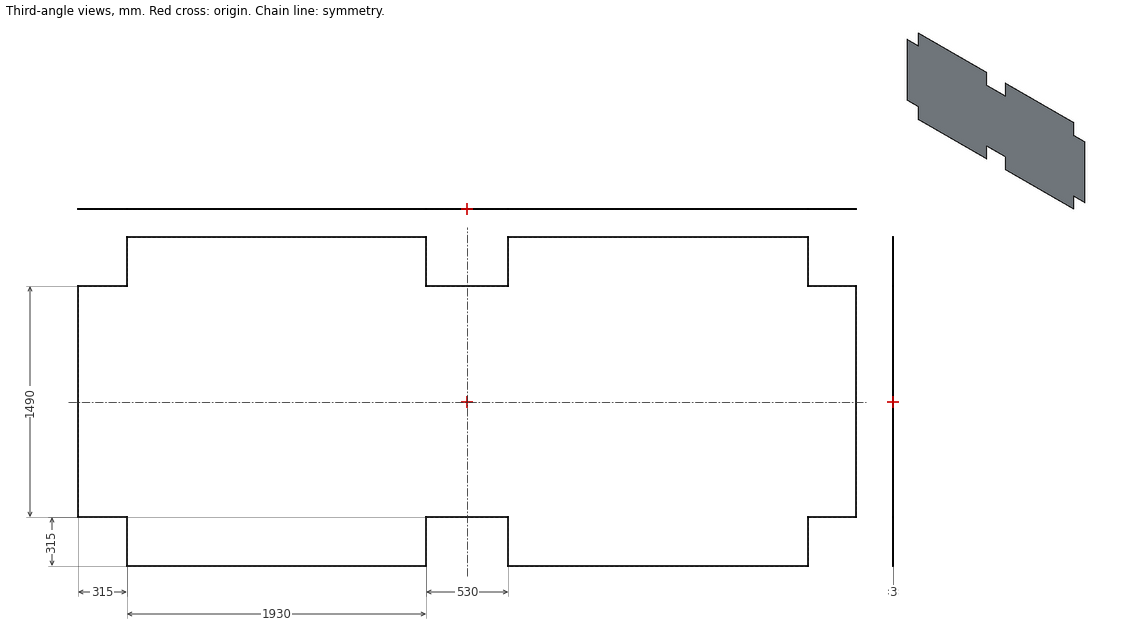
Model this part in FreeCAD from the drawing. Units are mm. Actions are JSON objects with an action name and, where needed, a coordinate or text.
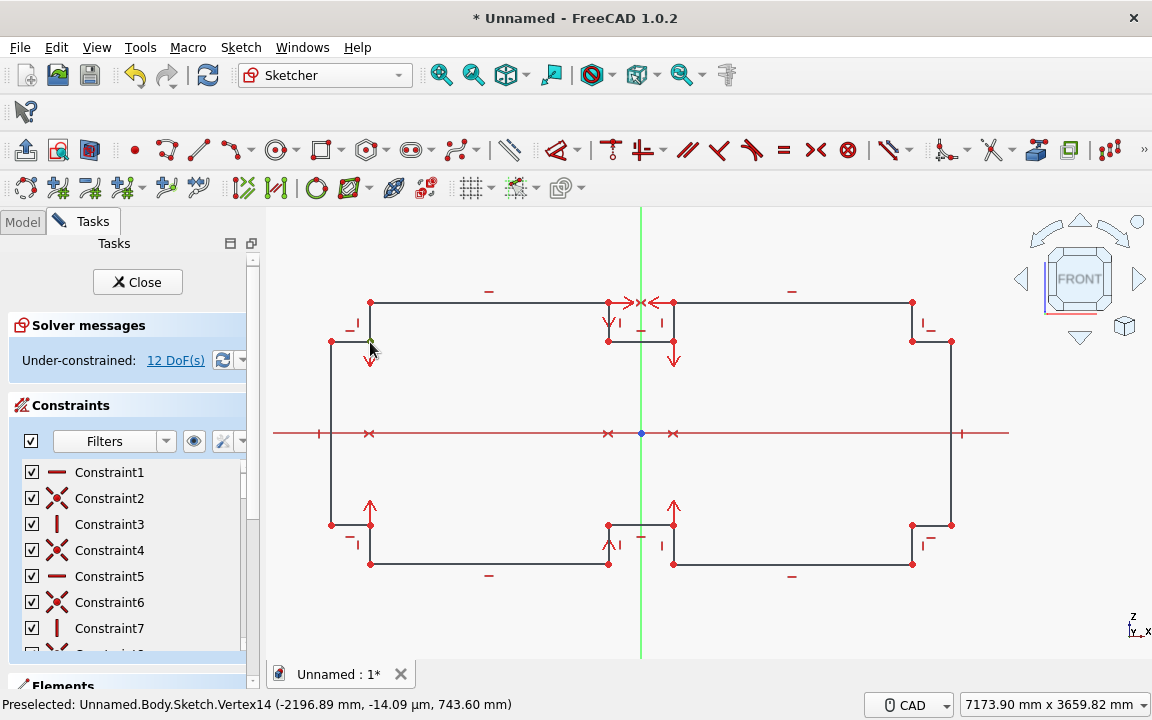
{"action": "left_click", "coordinate": [912, 342]}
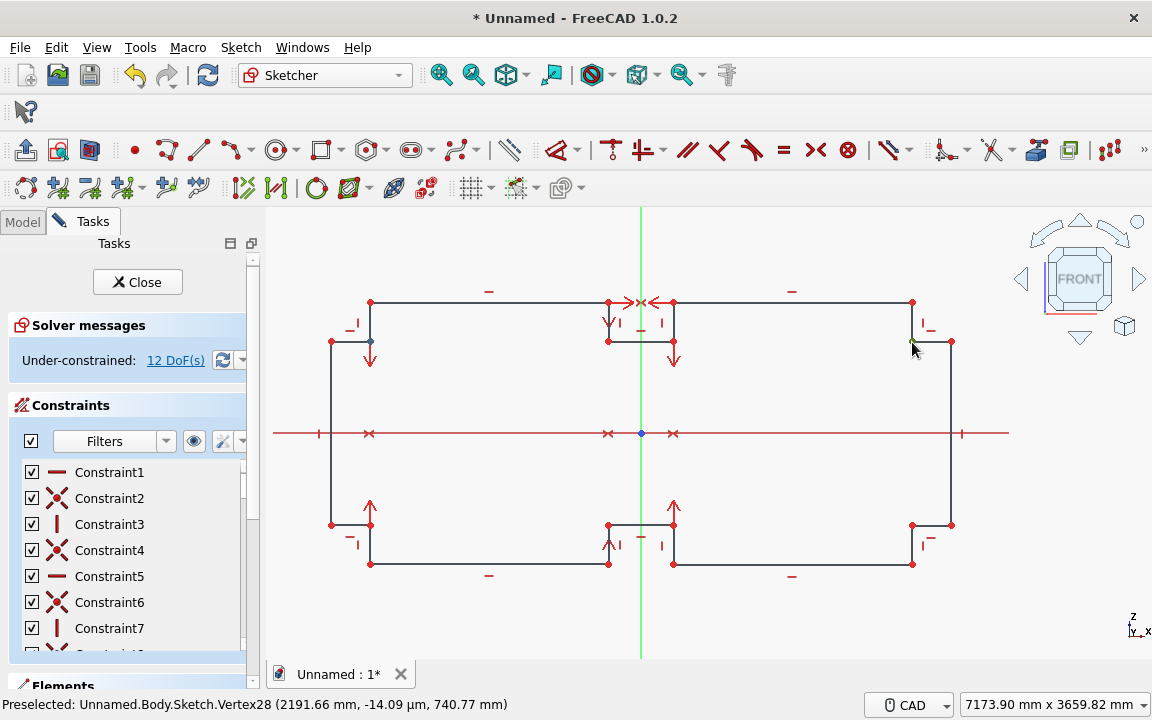
{"action": "left_click", "coordinate": [641, 603]}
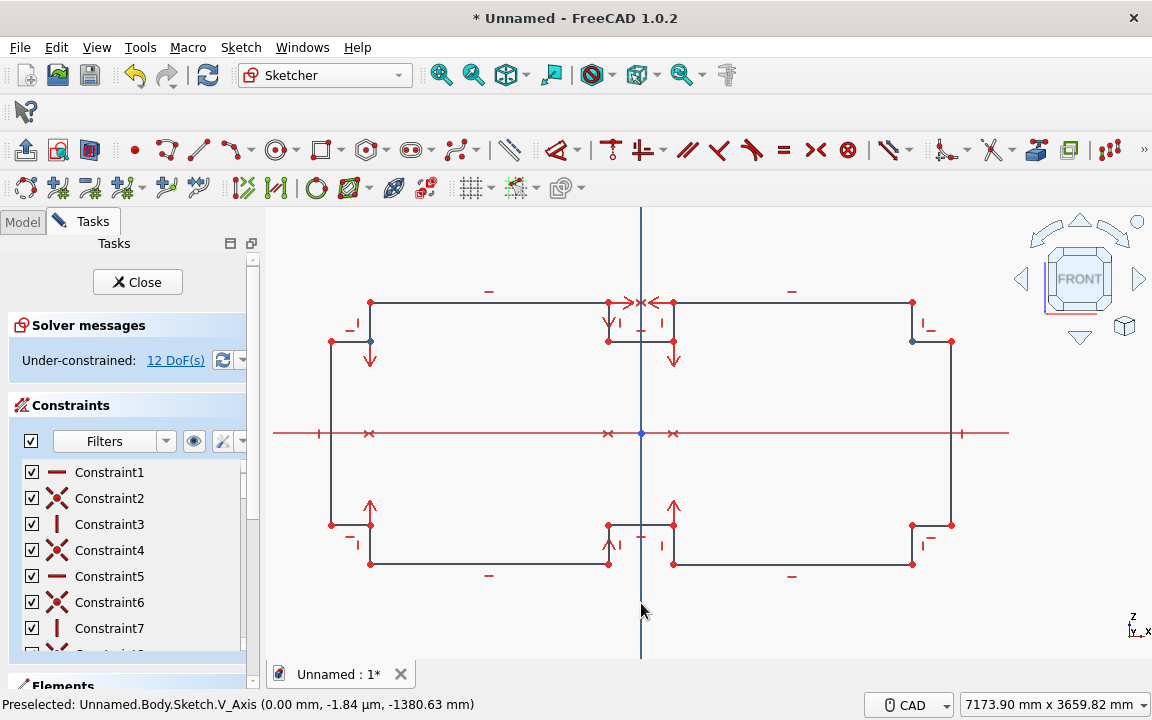
{"action": "left_click", "coordinate": [816, 150]}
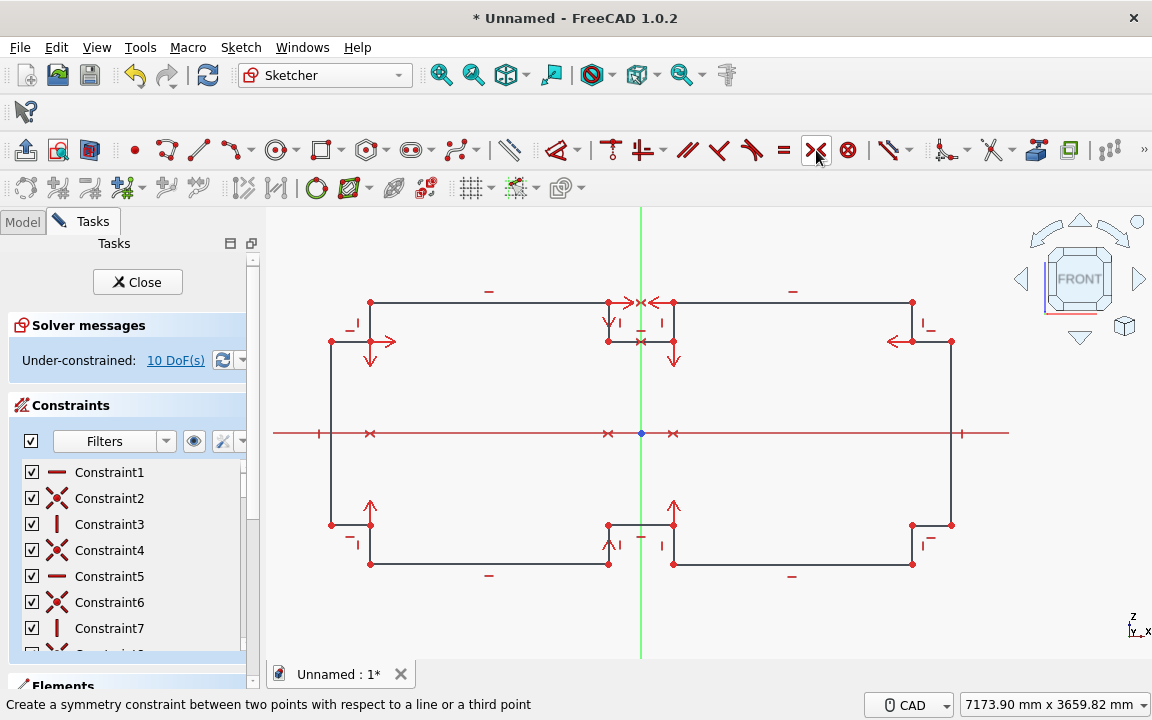
{"action": "left_click", "coordinate": [331, 525]}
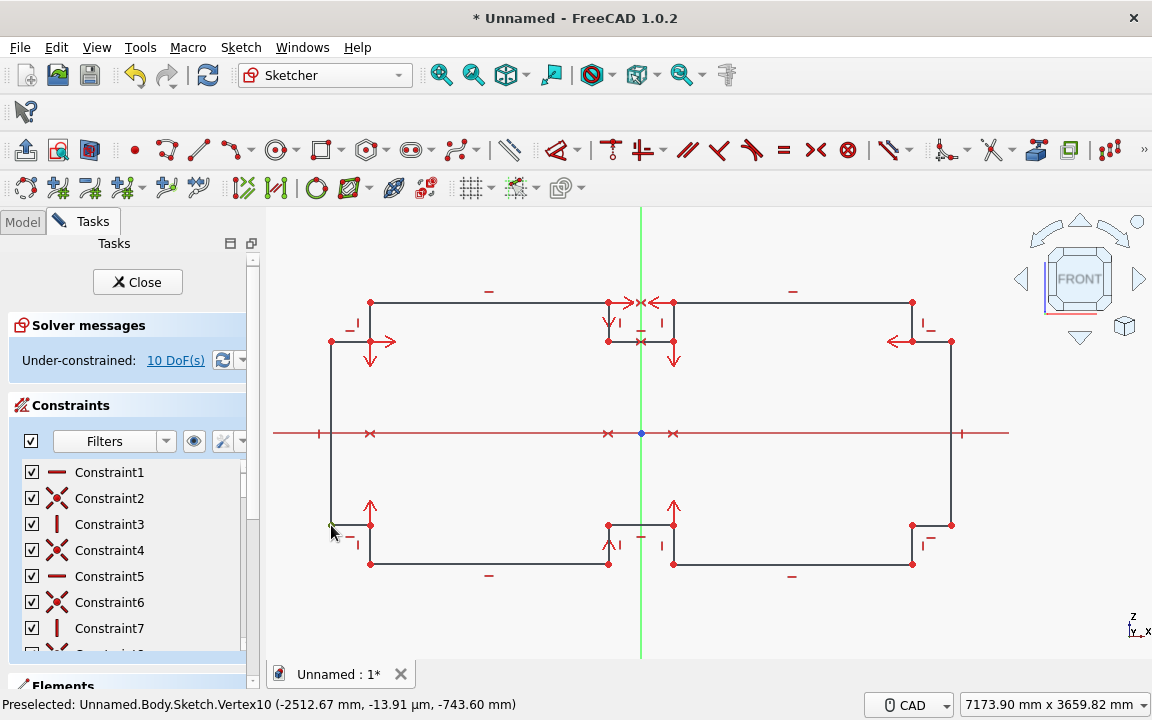
{"action": "left_click", "coordinate": [951, 526]}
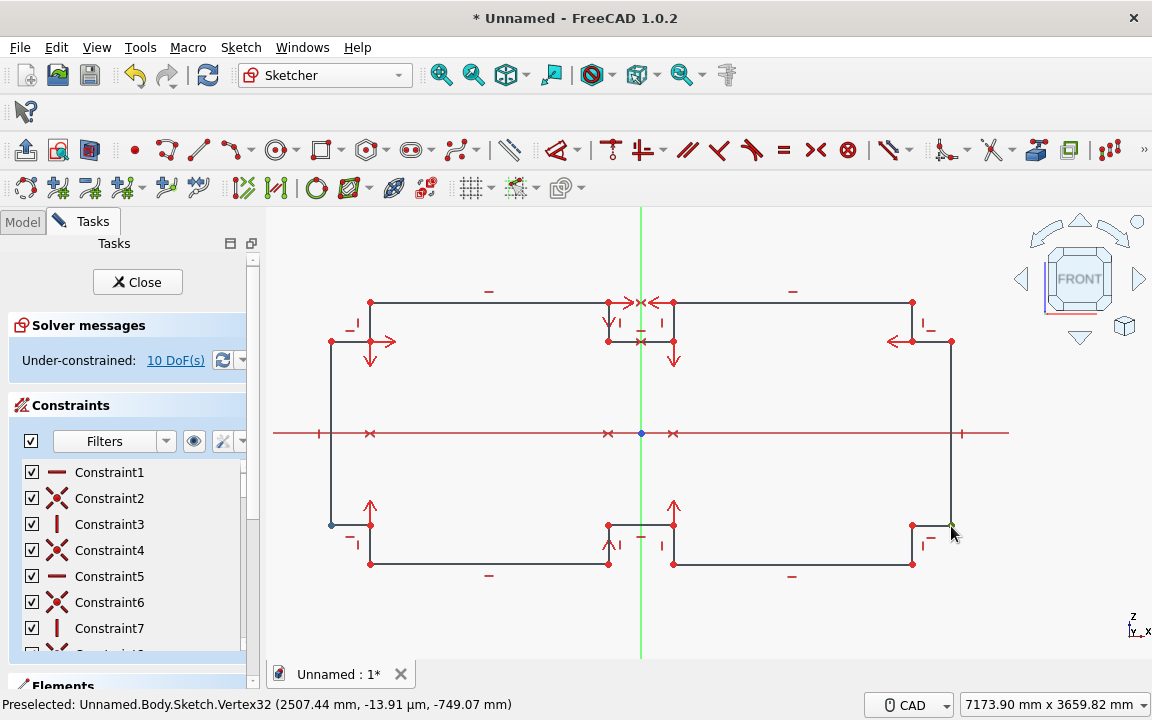
{"action": "left_click", "coordinate": [641, 603]}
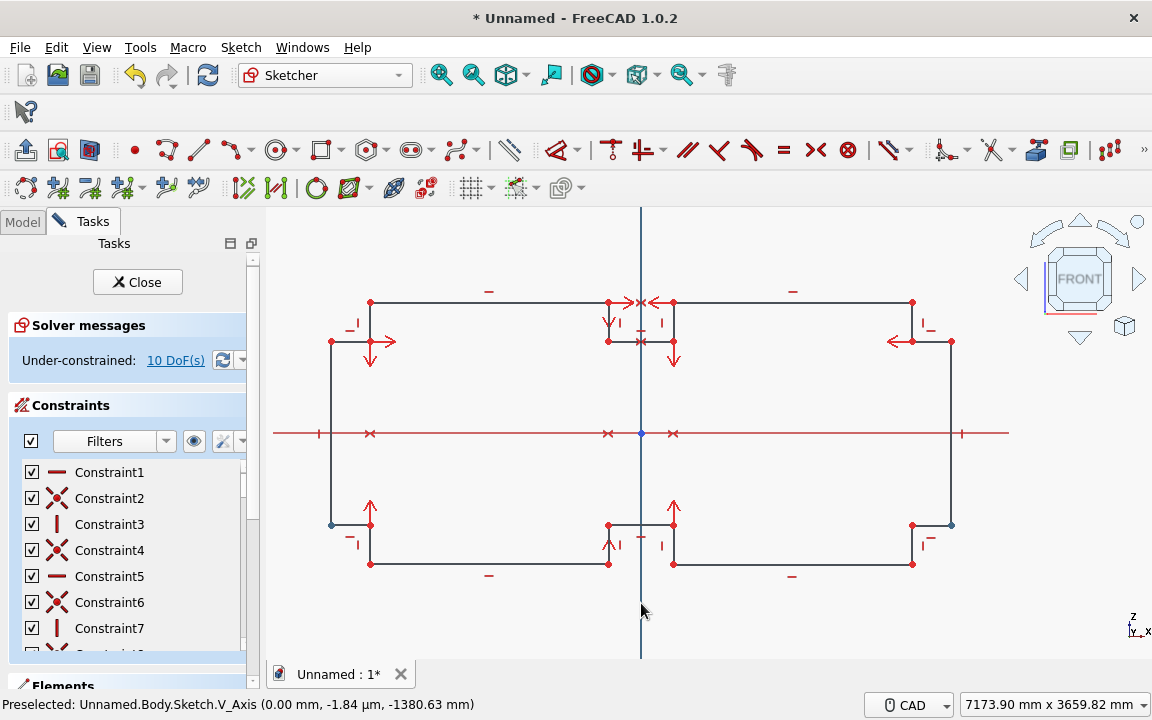
{"action": "left_click", "coordinate": [816, 150]}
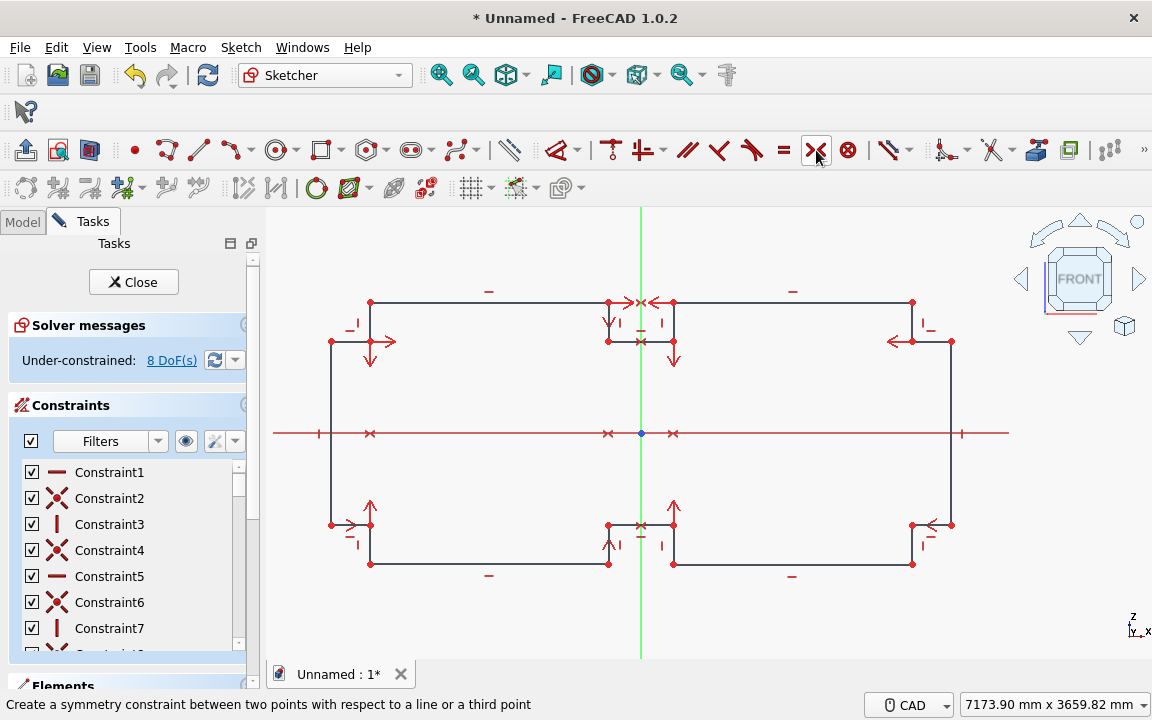
{"action": "left_click", "coordinate": [370, 564]}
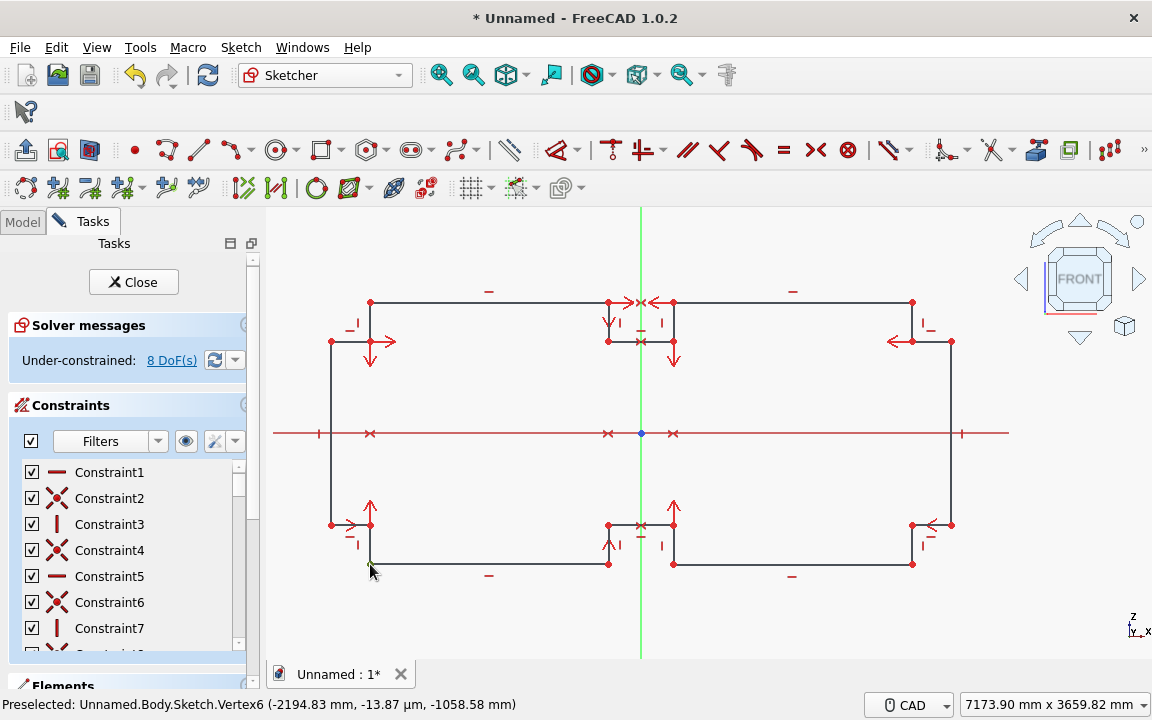
{"action": "left_click", "coordinate": [912, 565]}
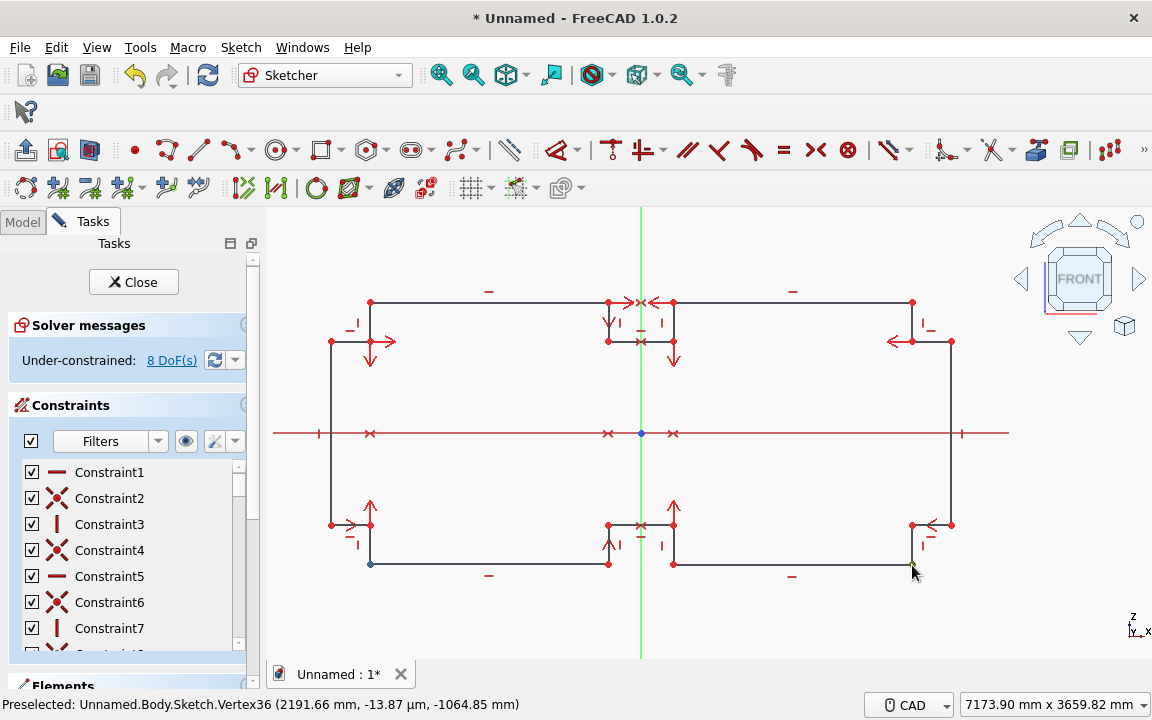
{"action": "left_click", "coordinate": [641, 603]}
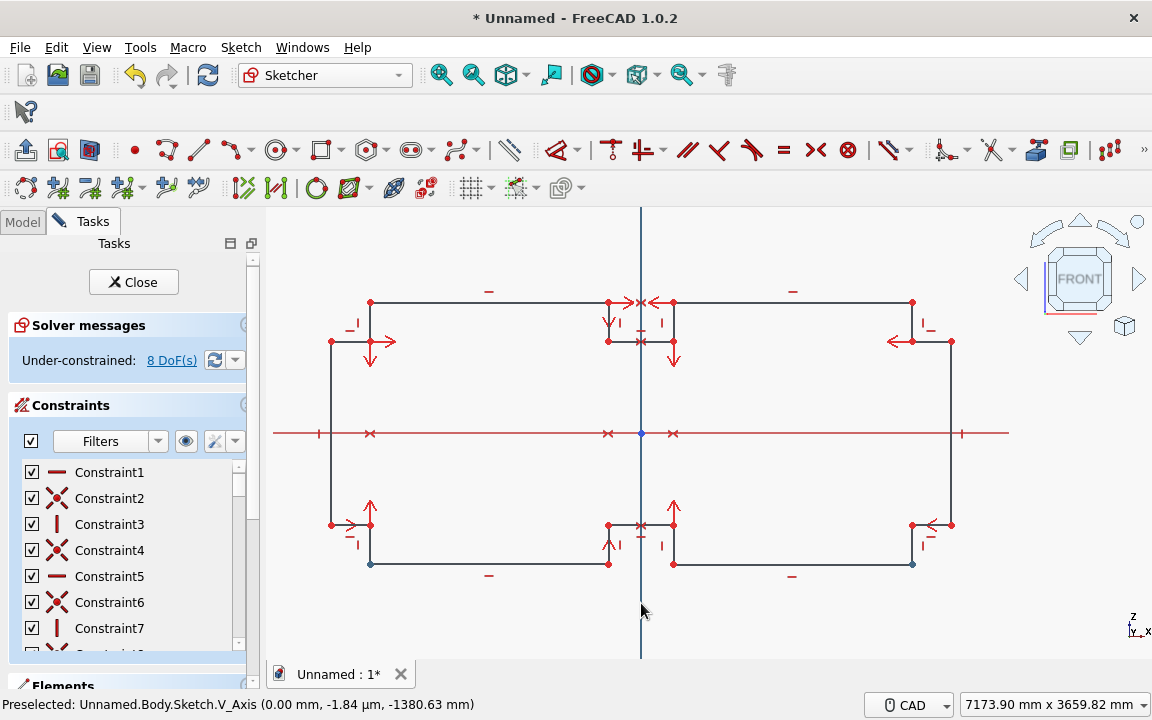
{"action": "left_click", "coordinate": [816, 150]}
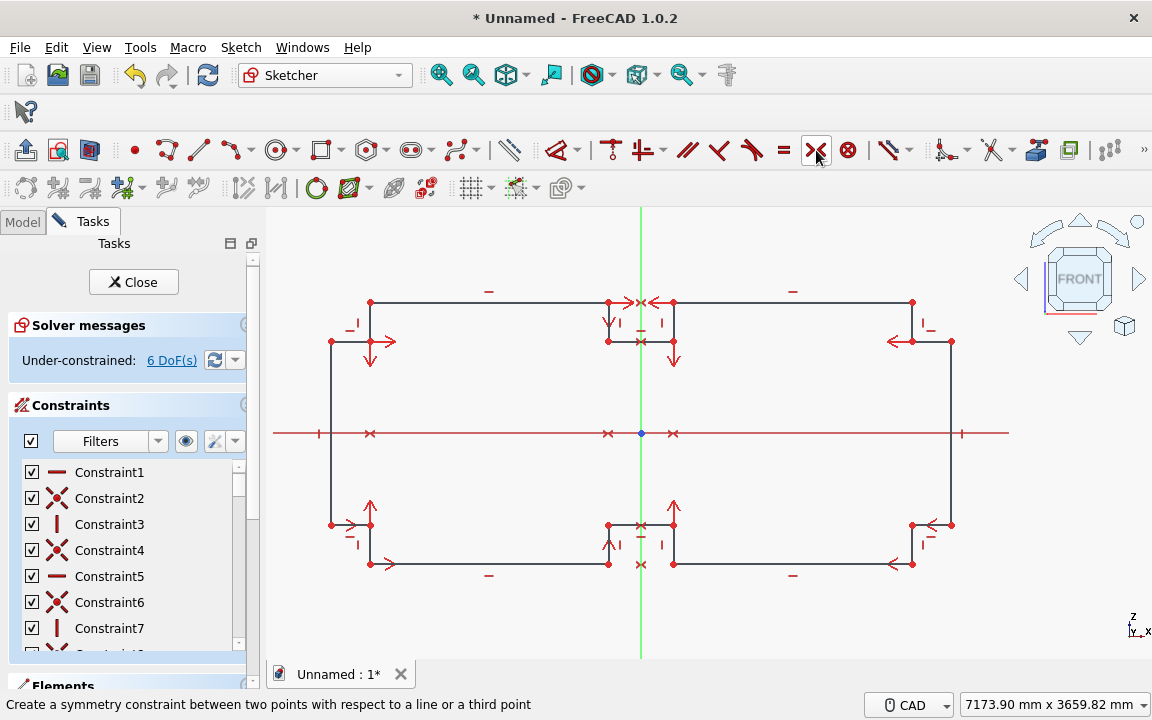
{"action": "left_click", "coordinate": [556, 150]}